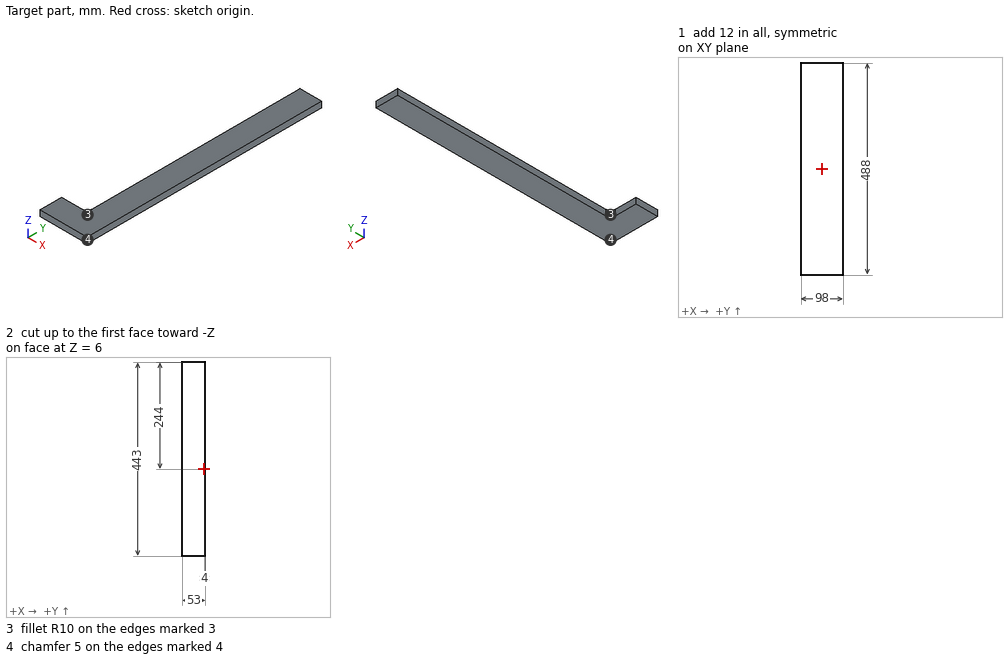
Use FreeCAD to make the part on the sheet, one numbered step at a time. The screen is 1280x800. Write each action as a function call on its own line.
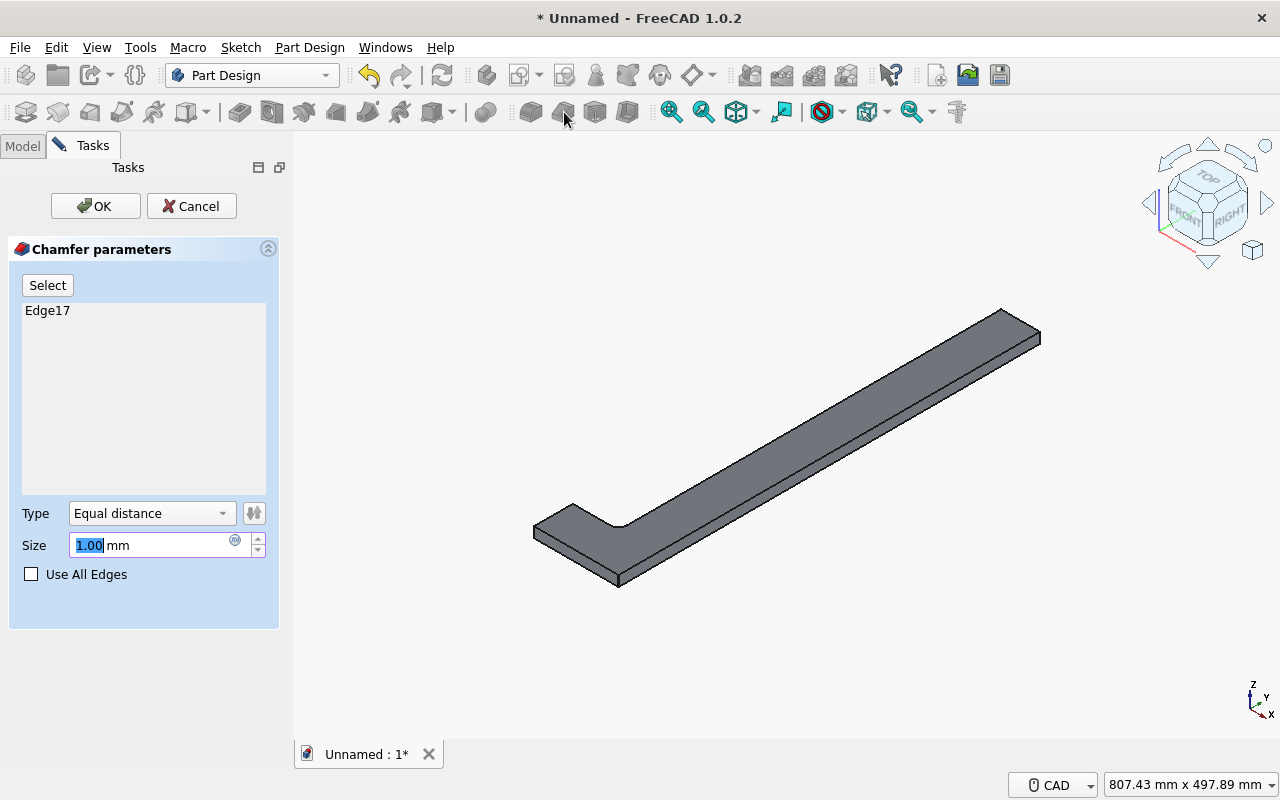
text(5)
key(Tab)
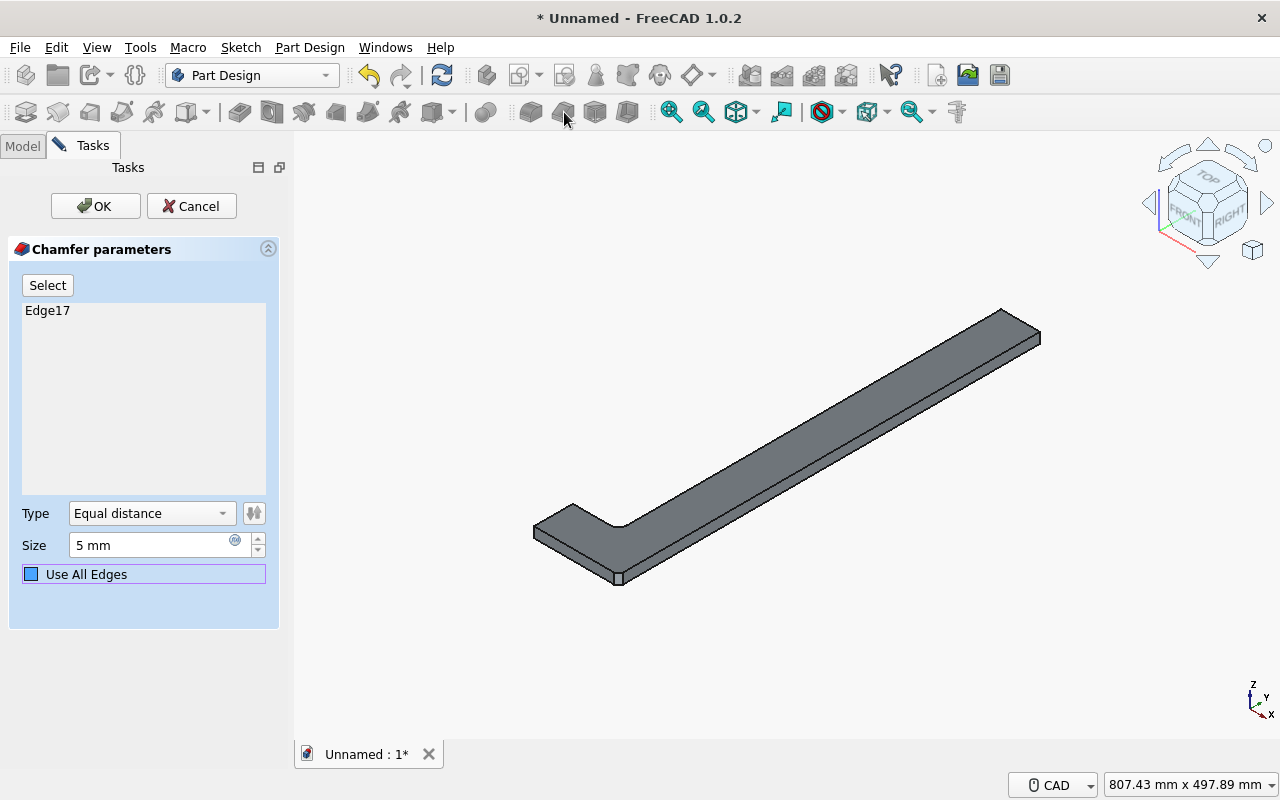
click(96, 206)